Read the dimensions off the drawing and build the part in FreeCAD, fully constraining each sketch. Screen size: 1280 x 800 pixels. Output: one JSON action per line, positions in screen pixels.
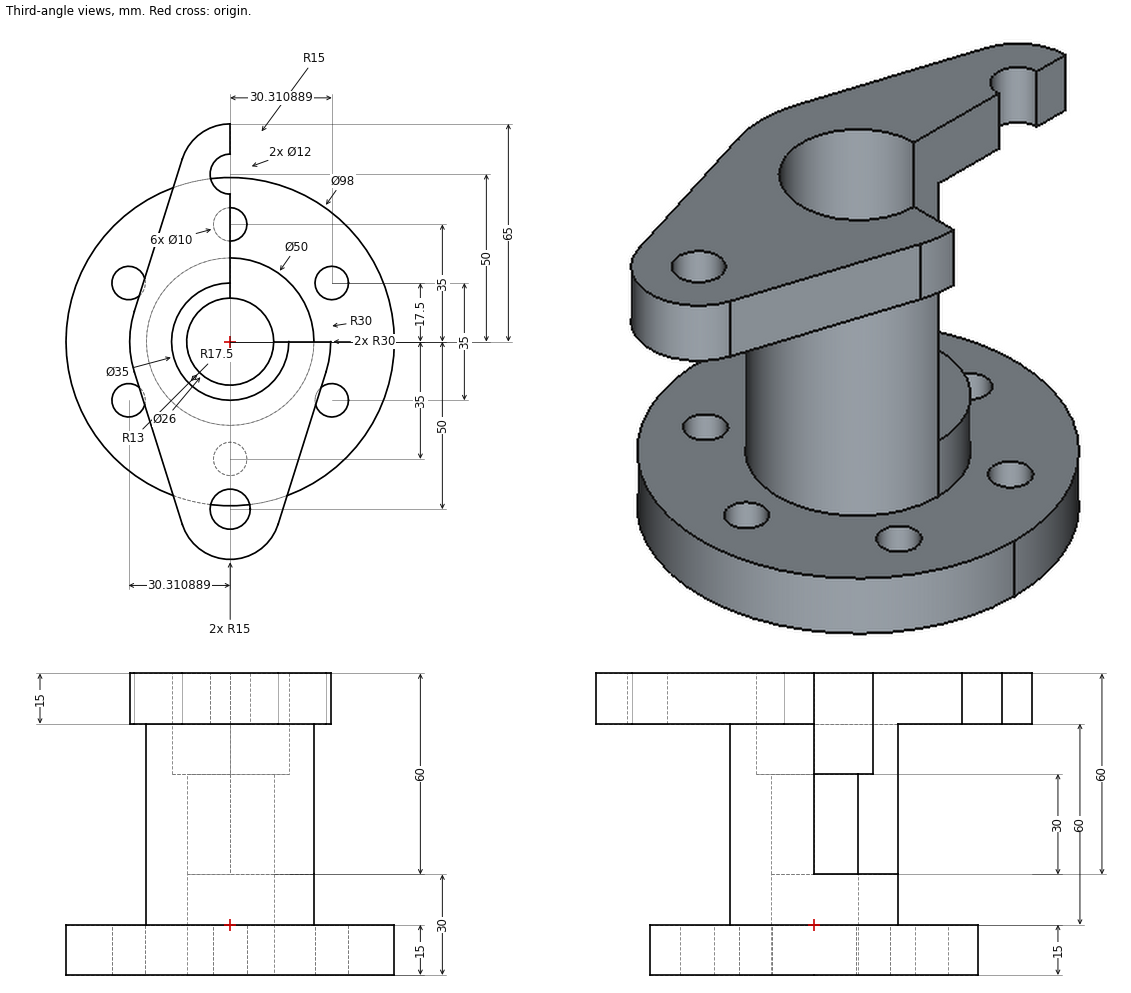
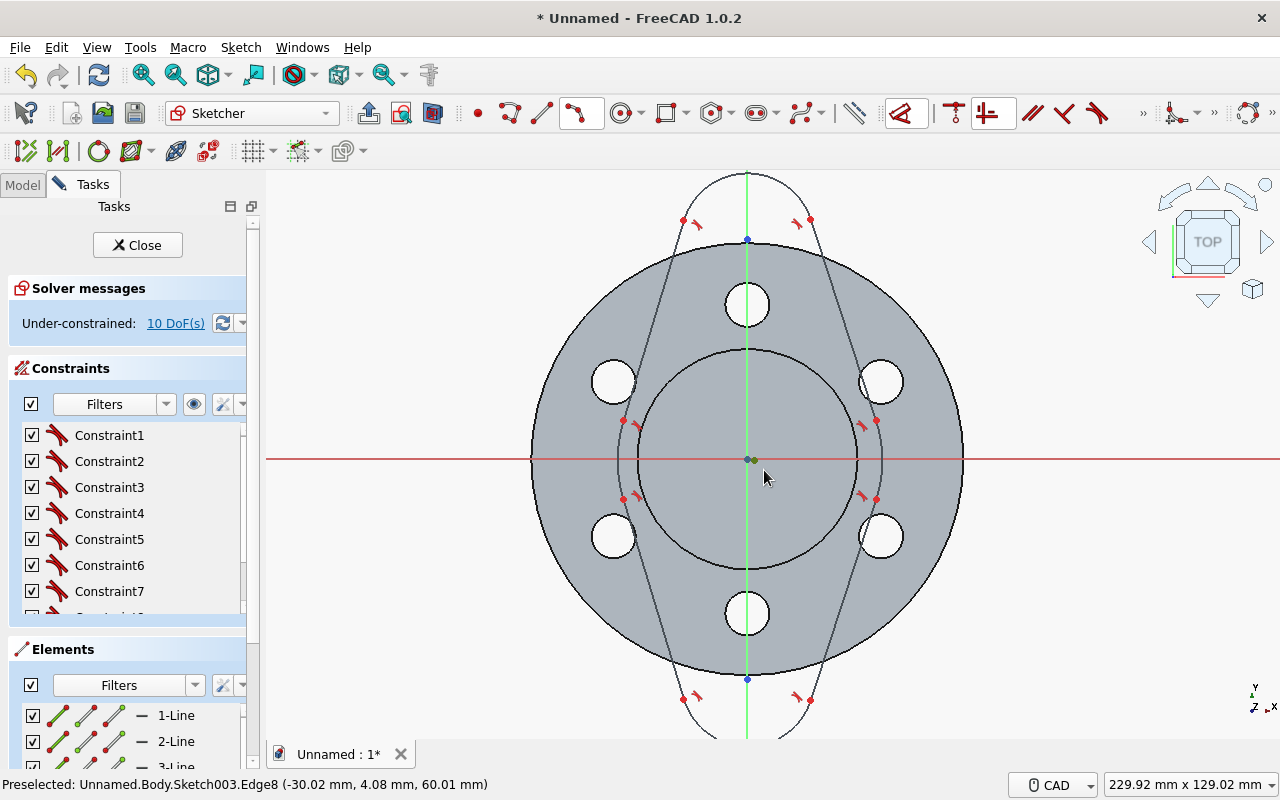
{"action": "key", "text": "c"}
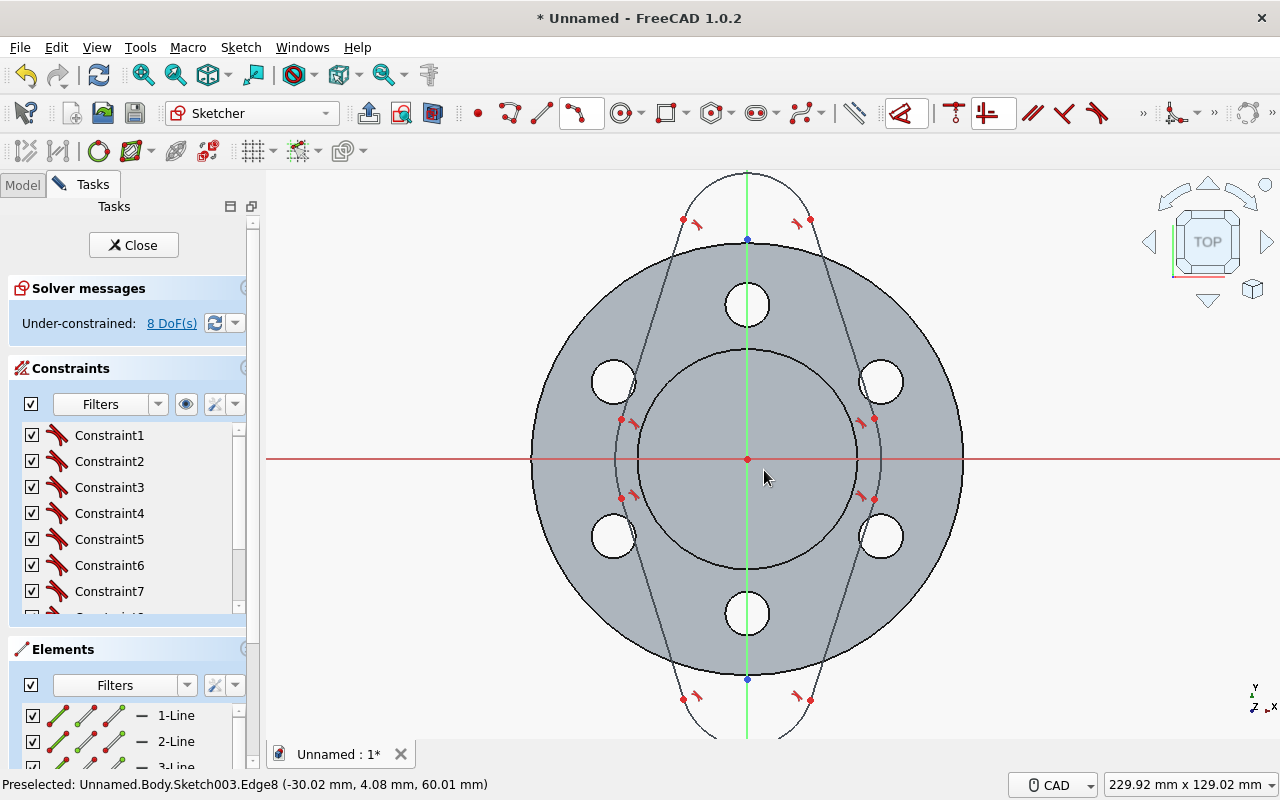
{"action": "scroll", "coordinate": [617, 445], "scroll_direction": "down", "scroll_amount": 2}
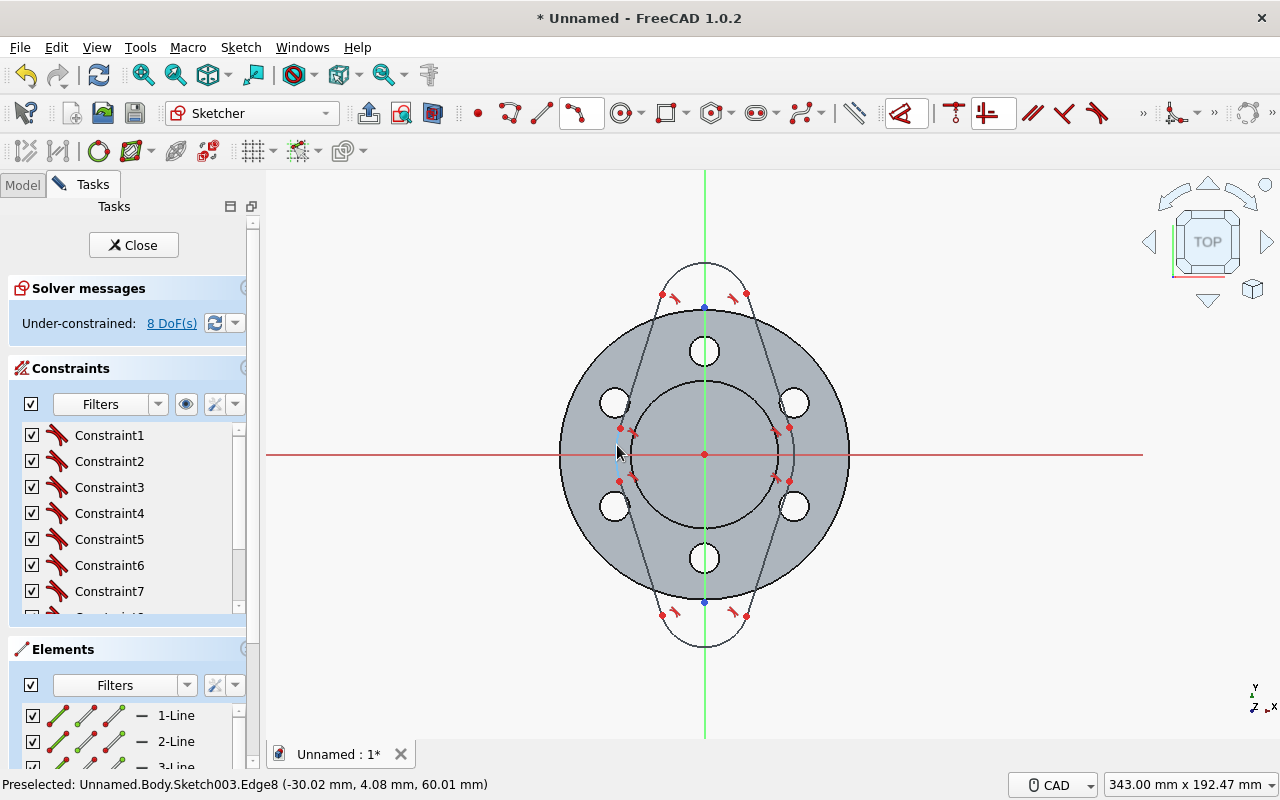
{"action": "left_click", "coordinate": [683, 642]}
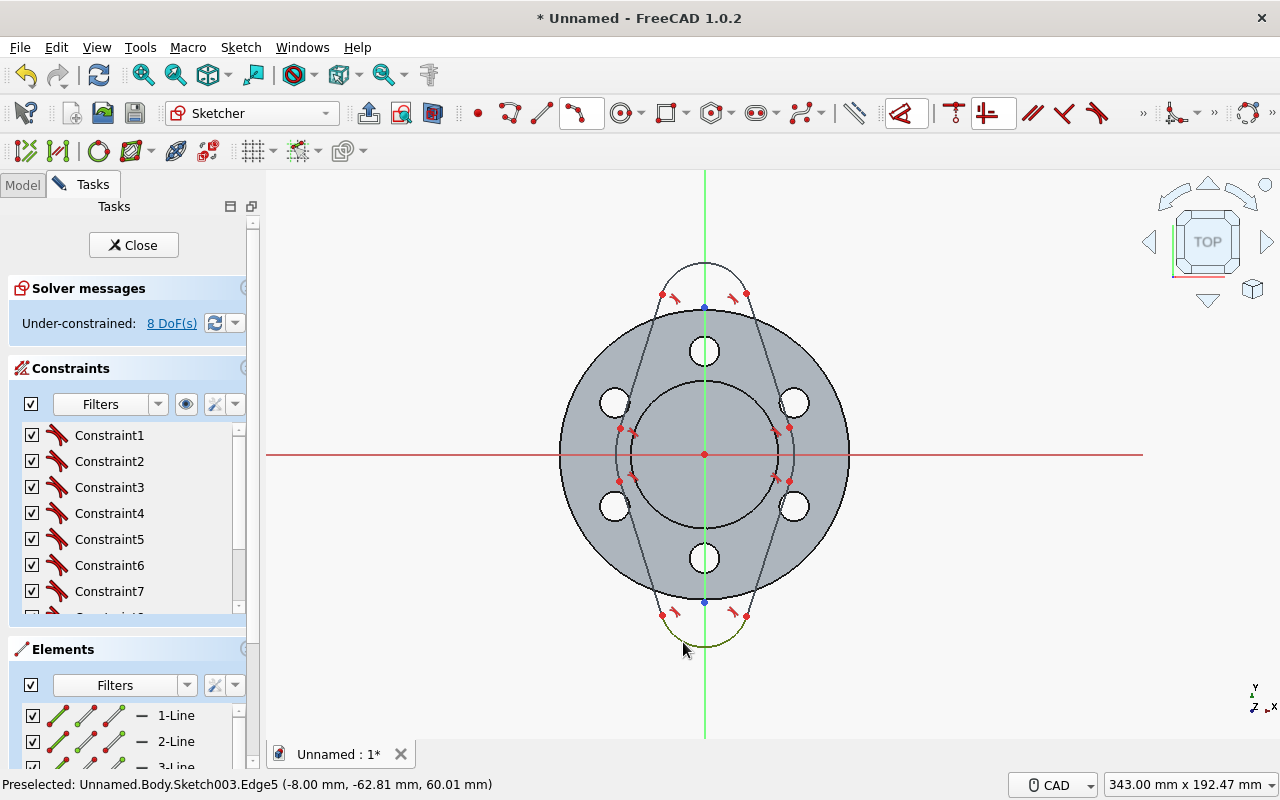
{"action": "left_click", "coordinate": [726, 269]}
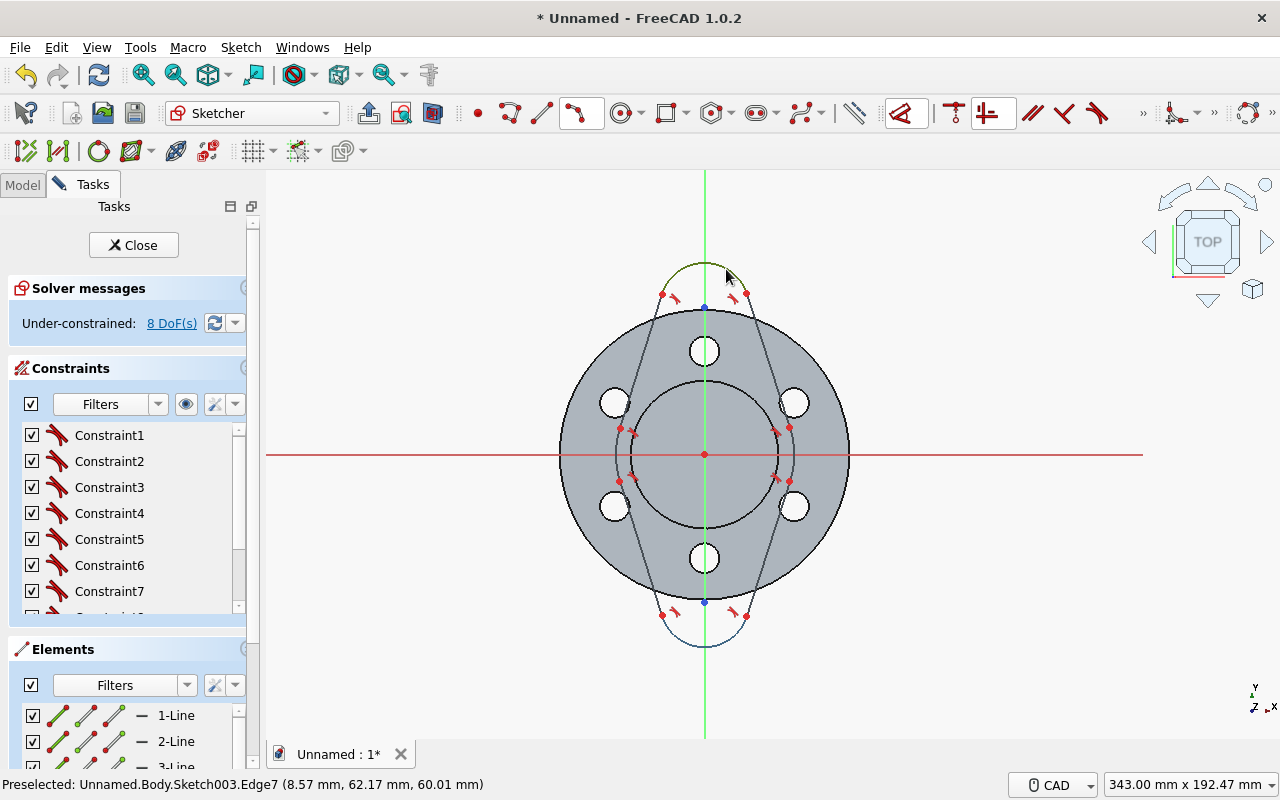
{"action": "key", "text": "e"}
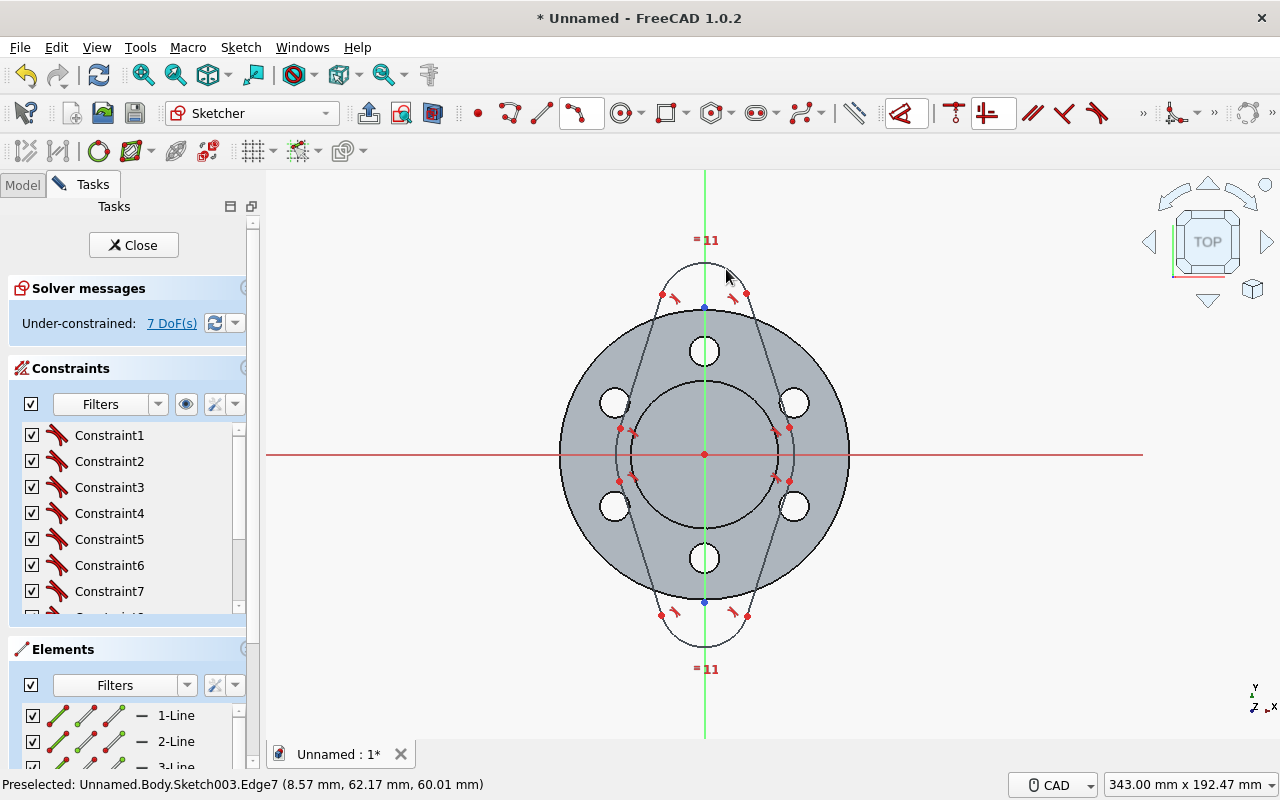
{"action": "scroll", "coordinate": [793, 466], "scroll_direction": "up", "scroll_amount": 2}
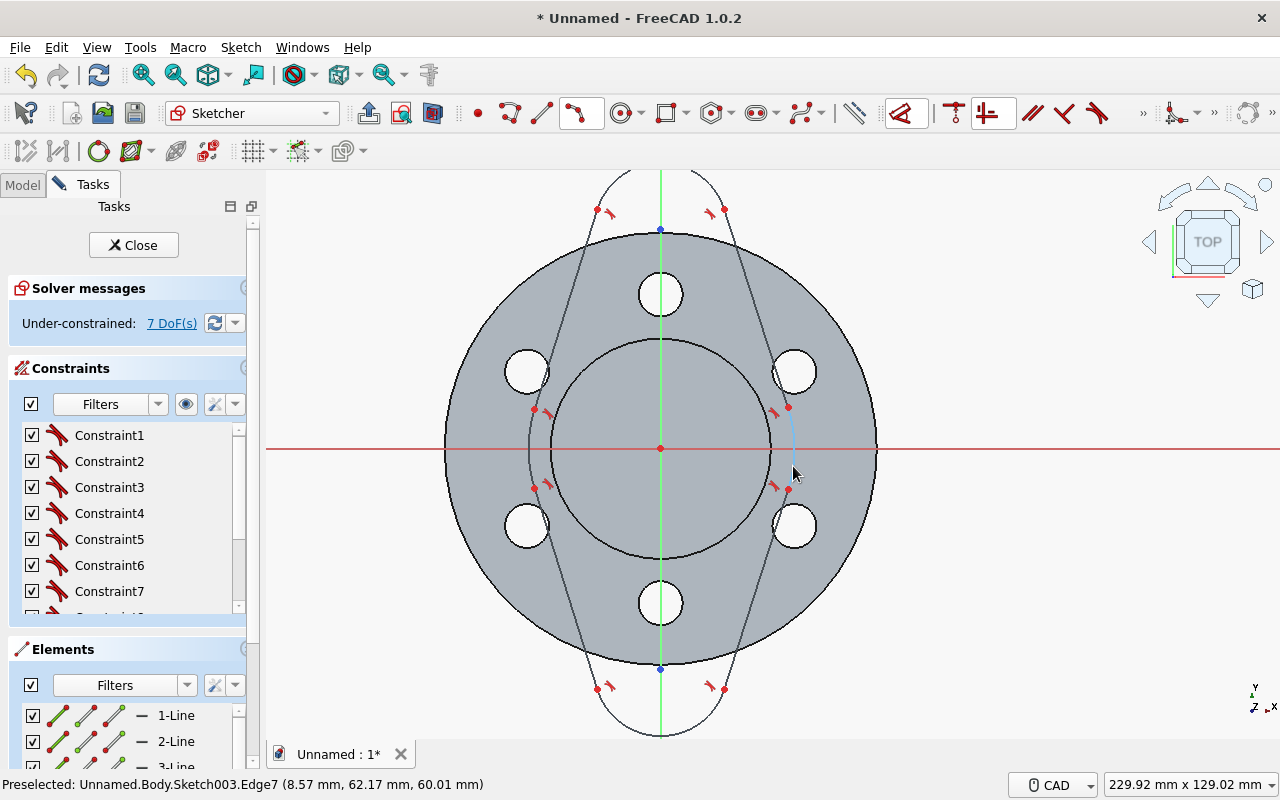
{"action": "left_click", "coordinate": [793, 465]}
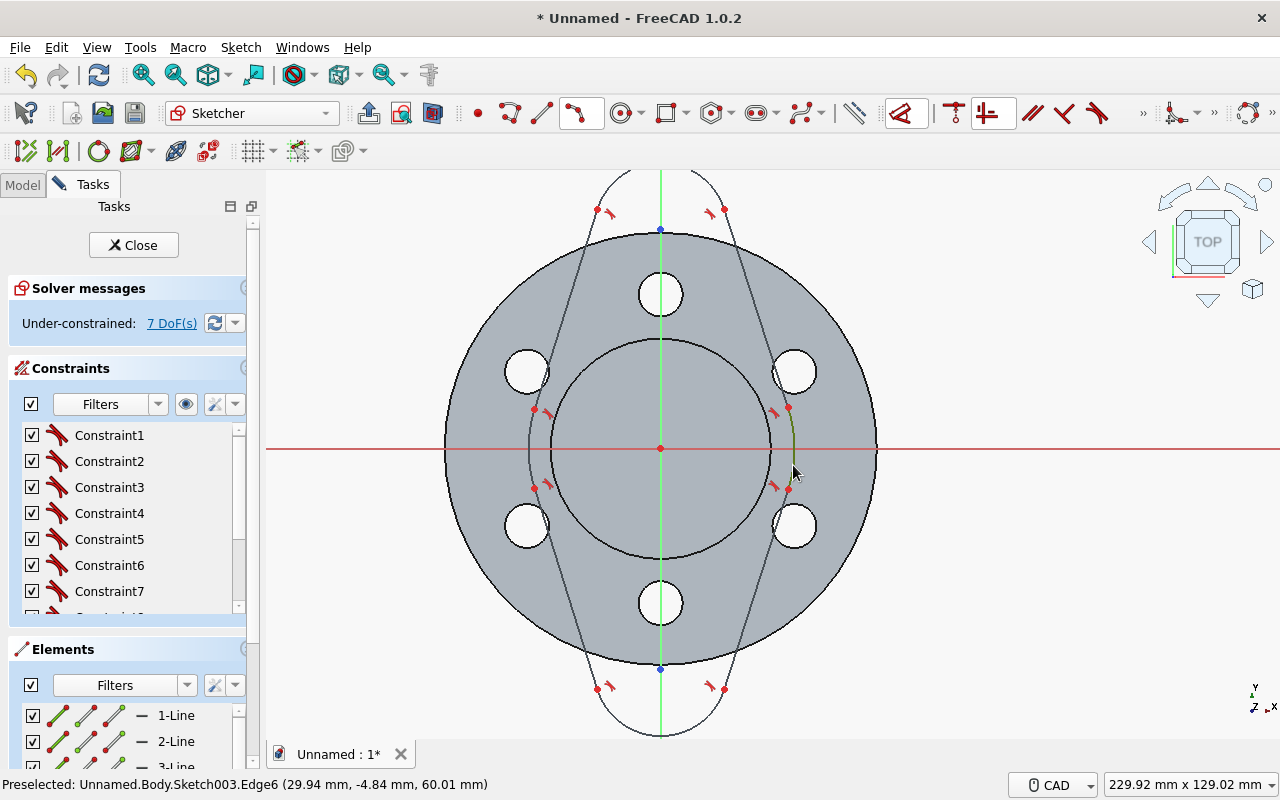
{"action": "left_click", "coordinate": [530, 433]}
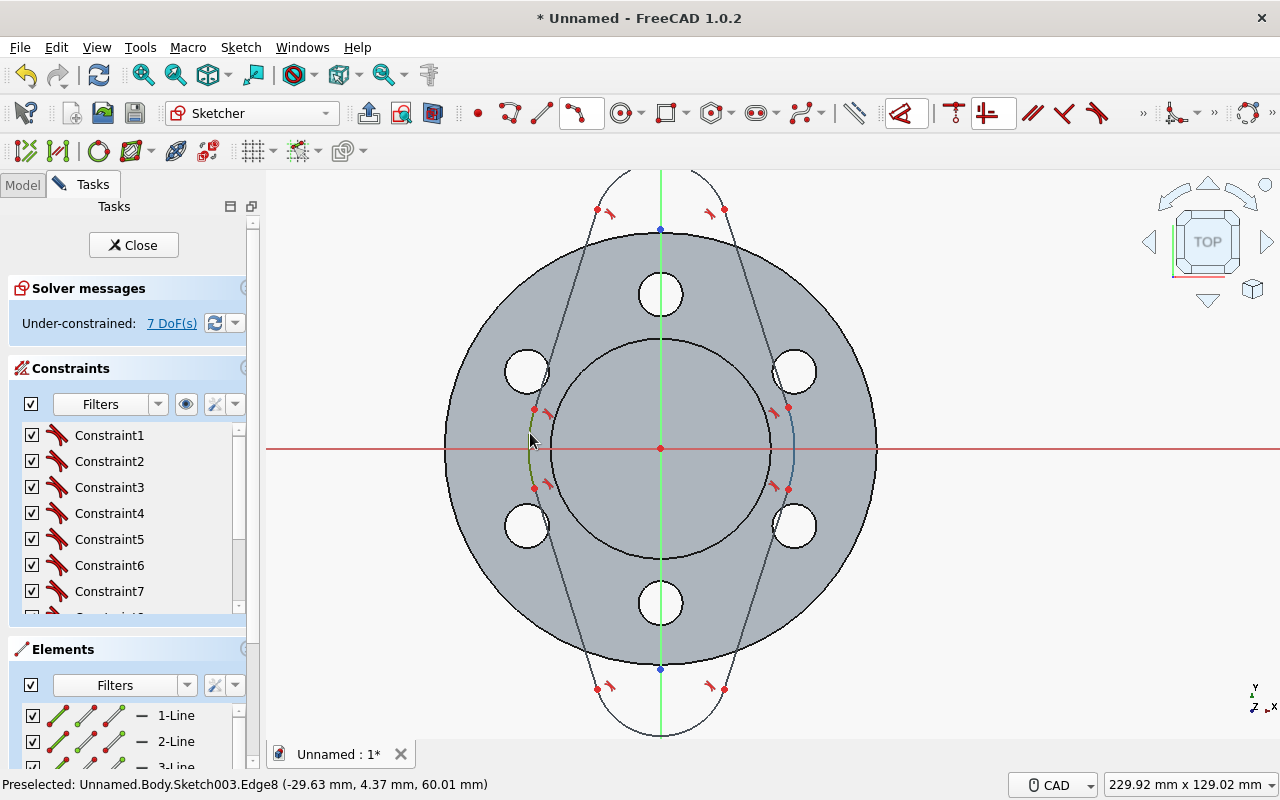
{"action": "key", "text": "e"}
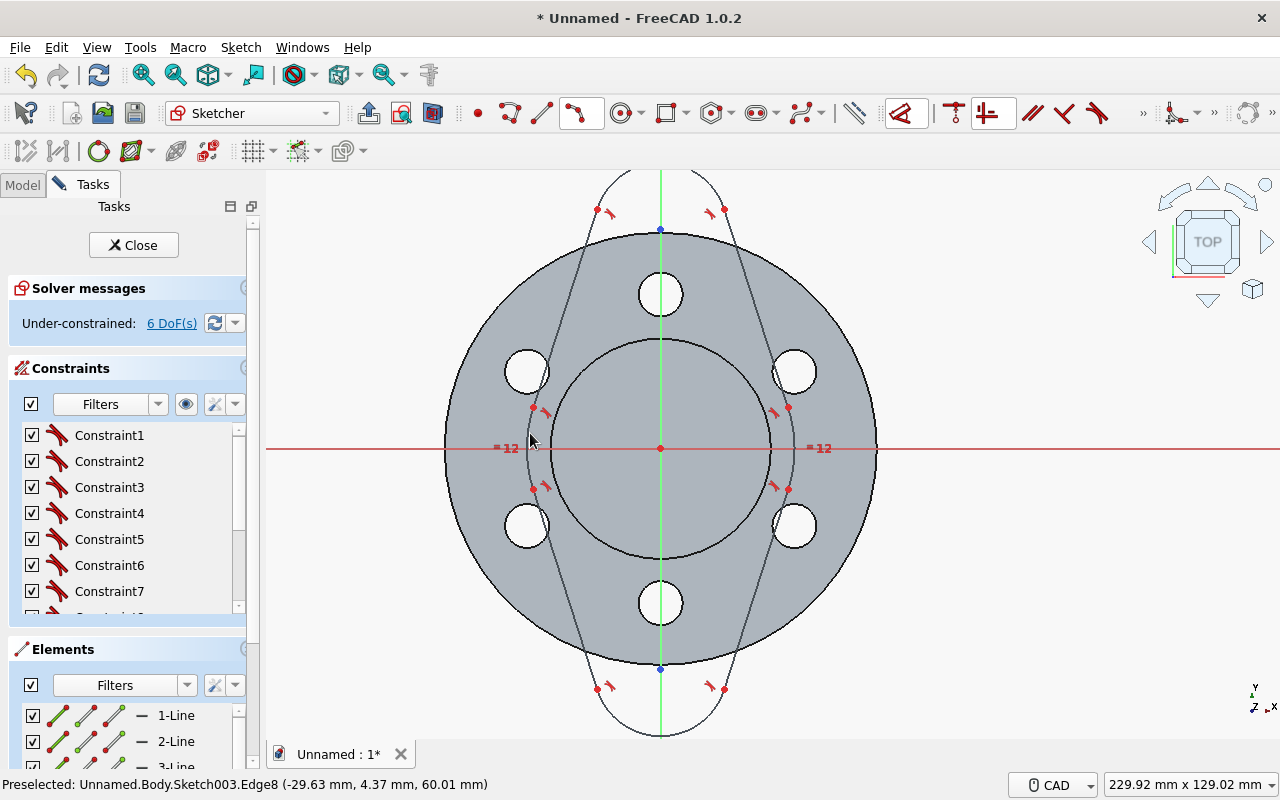
{"action": "left_click", "coordinate": [661, 670]}